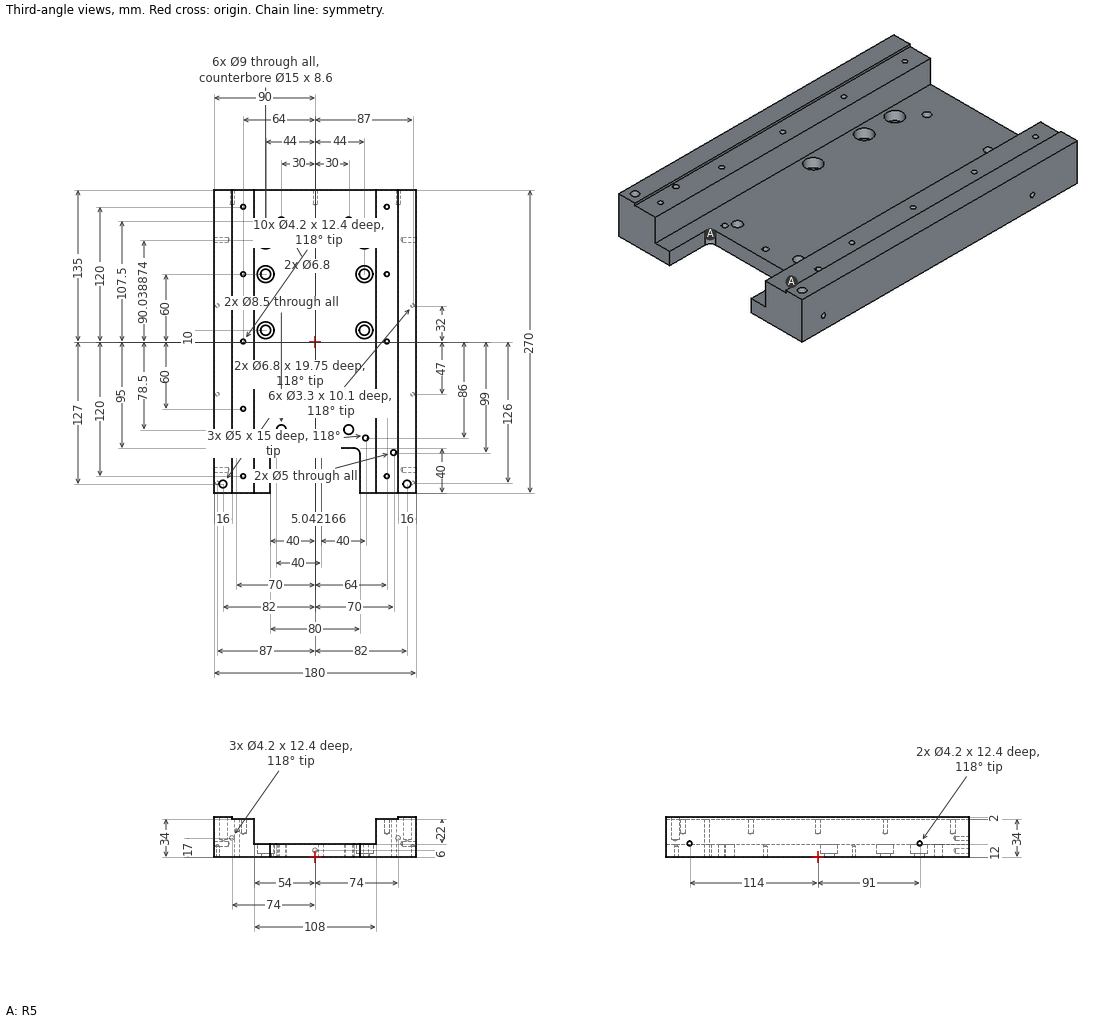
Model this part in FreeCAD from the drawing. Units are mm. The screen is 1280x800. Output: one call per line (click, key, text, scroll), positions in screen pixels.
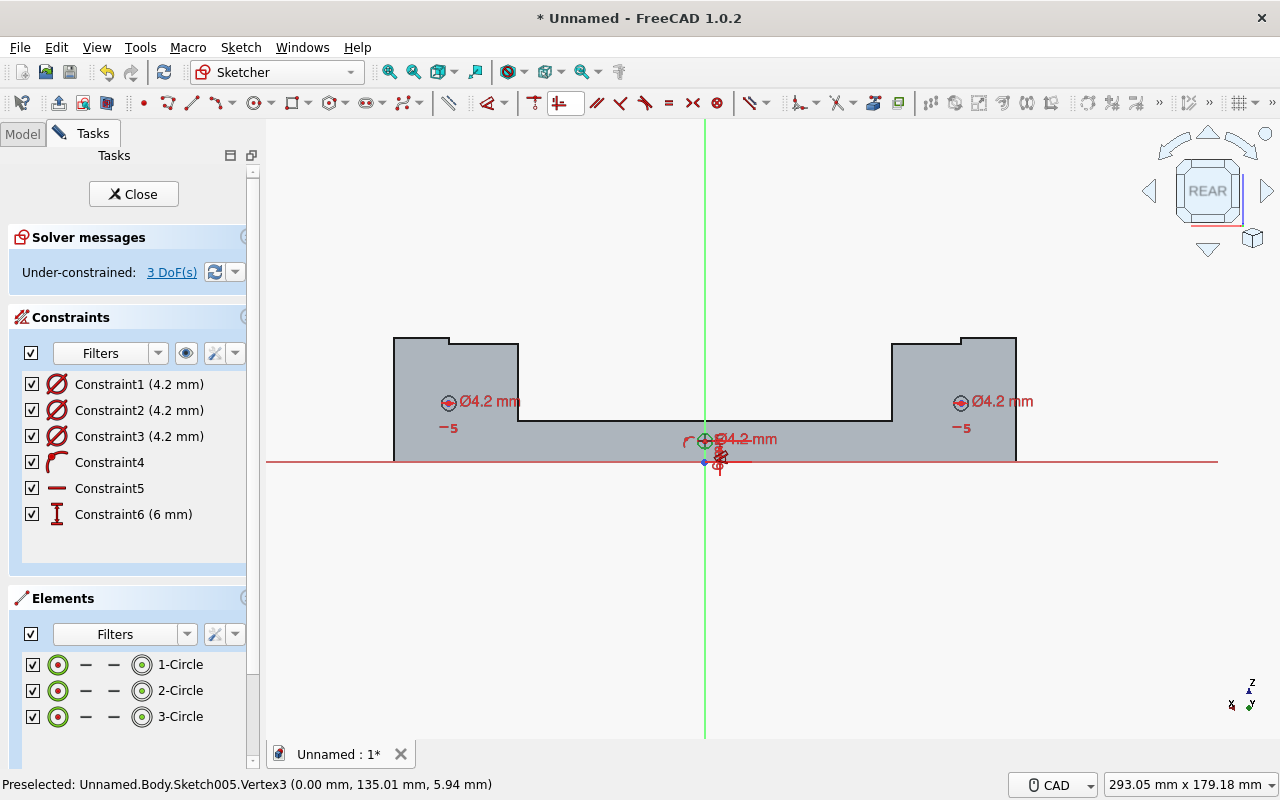
click(961, 403)
click(833, 496)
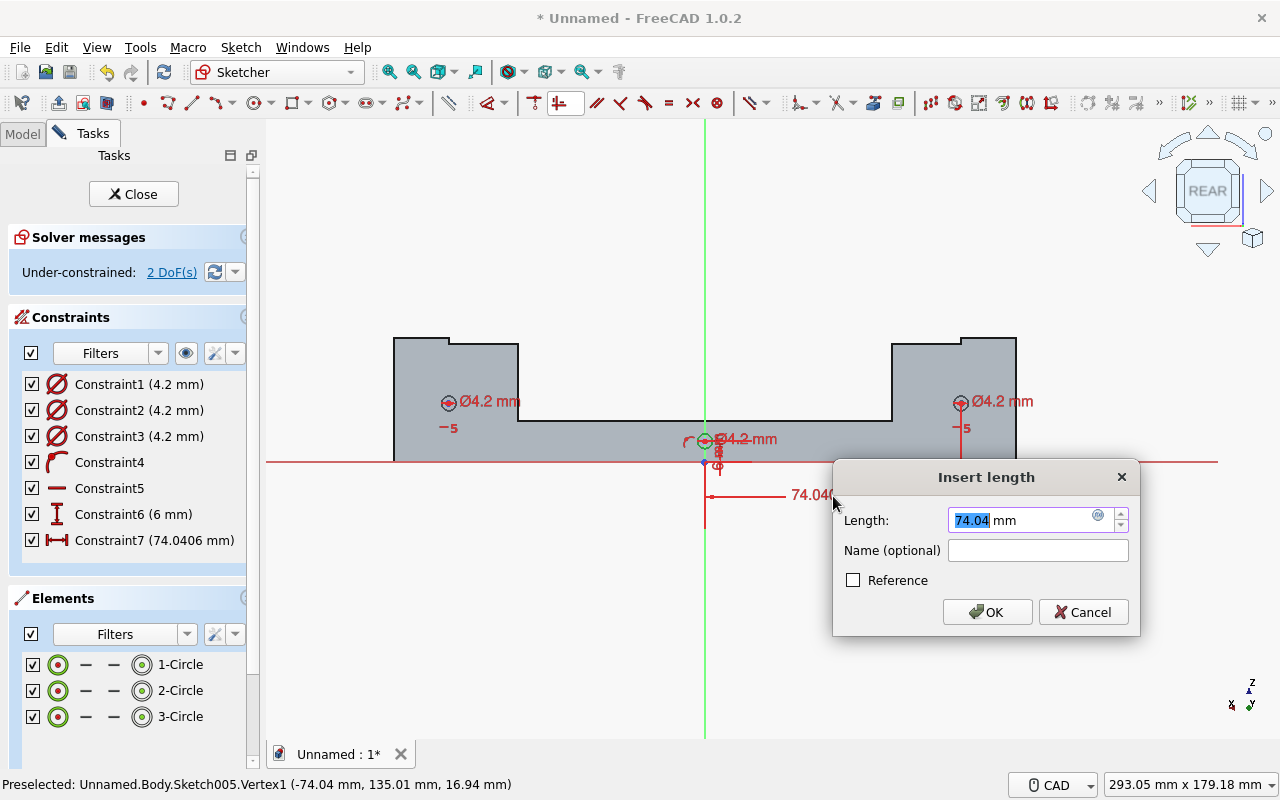
text(74)
key(Return)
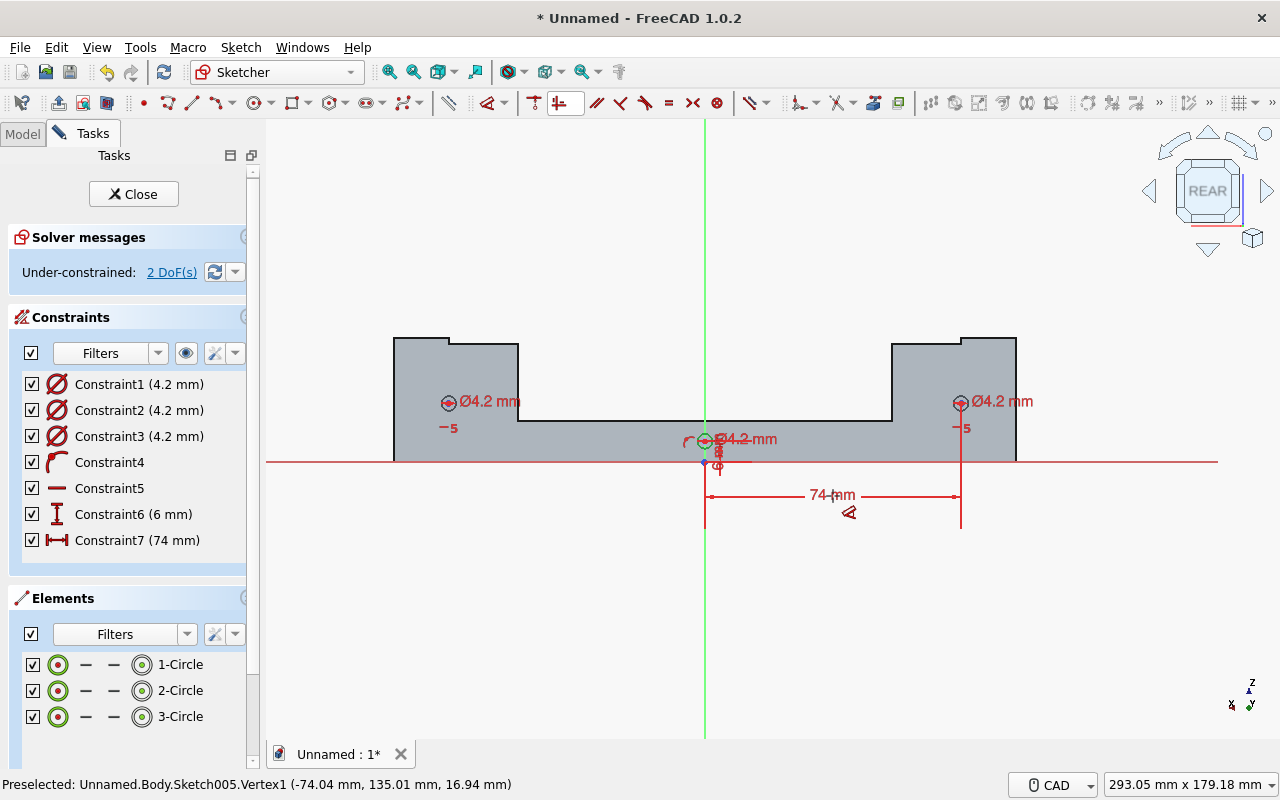
click(961, 403)
click(995, 433)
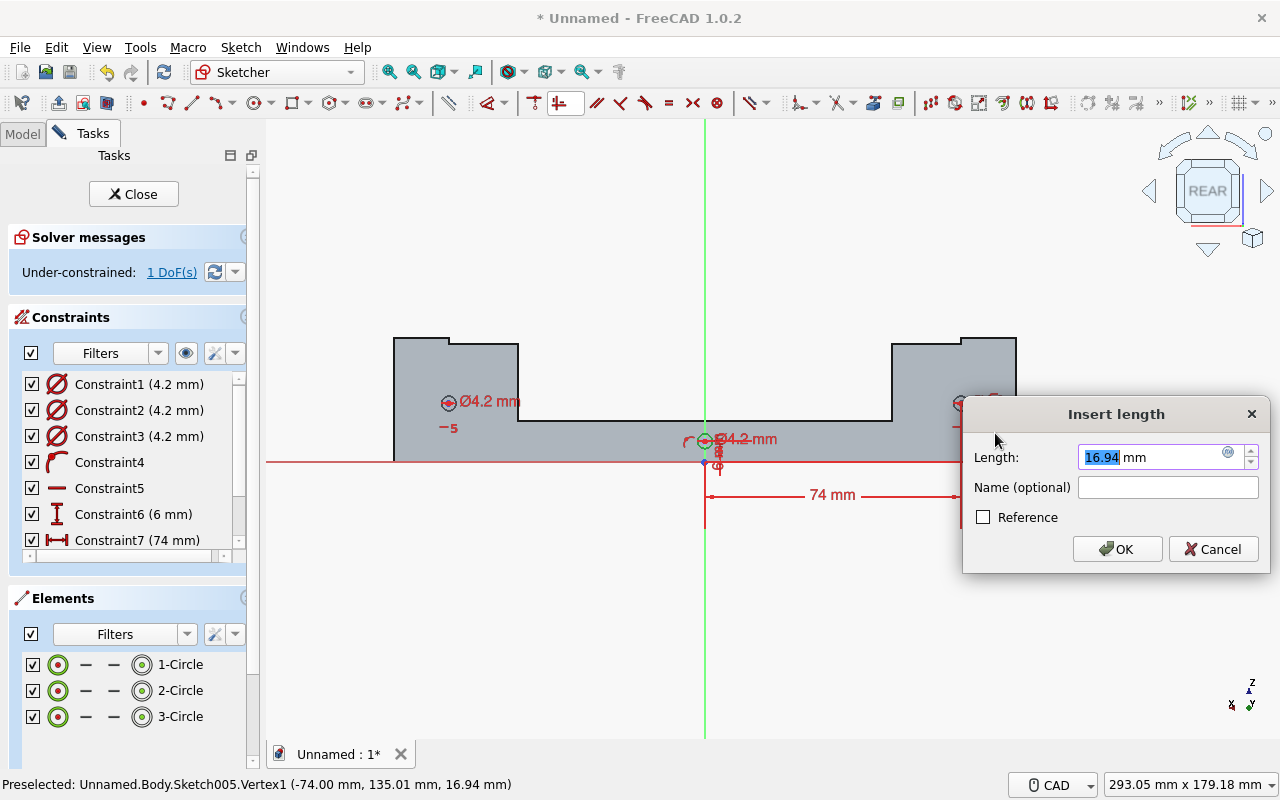
text(17)
key(Return)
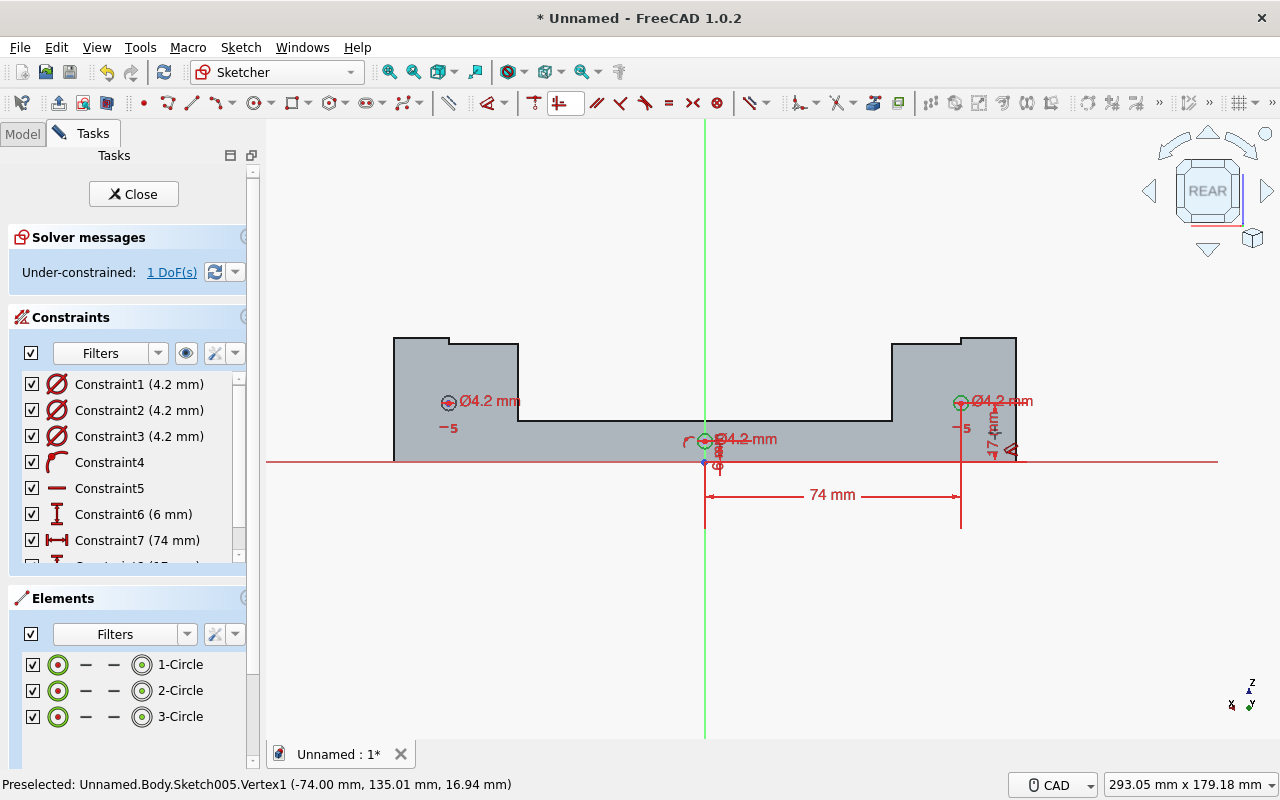
click(449, 403)
click(577, 496)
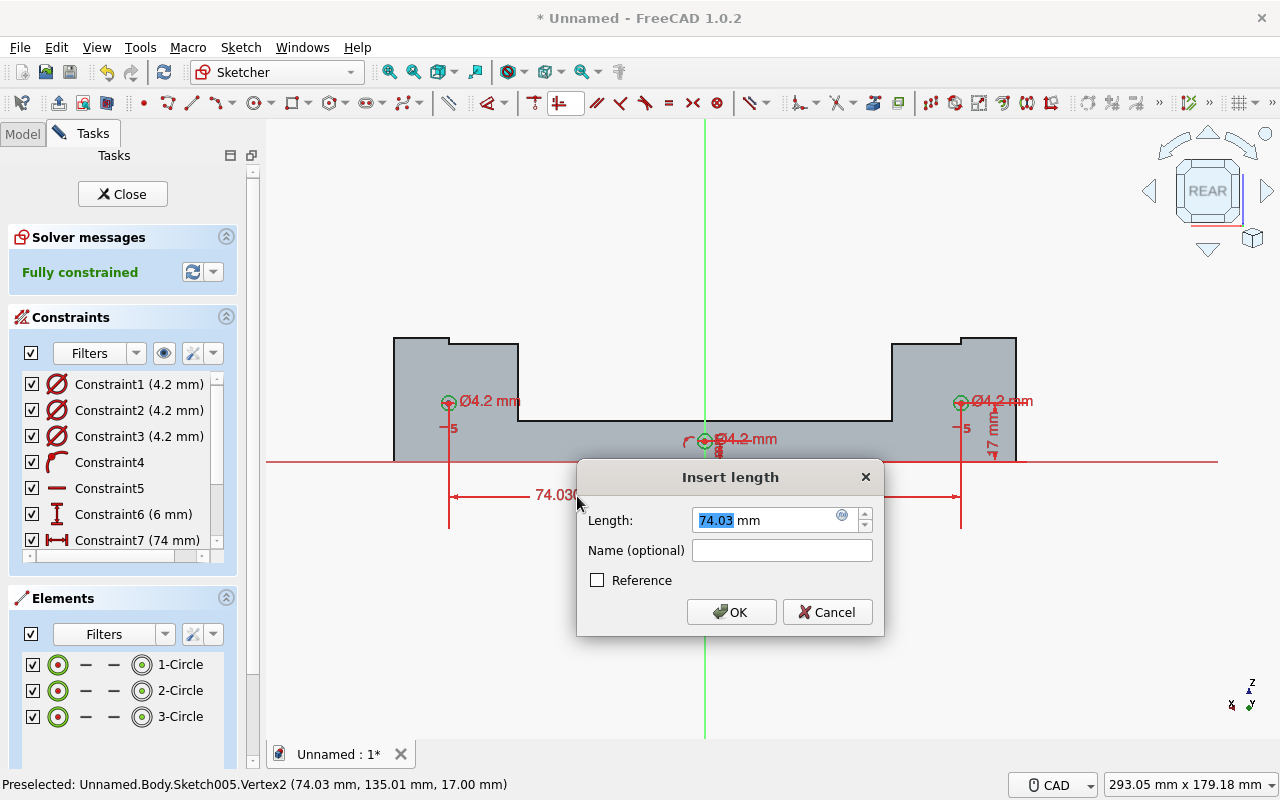
text(74)
key(Return)
key(Escape)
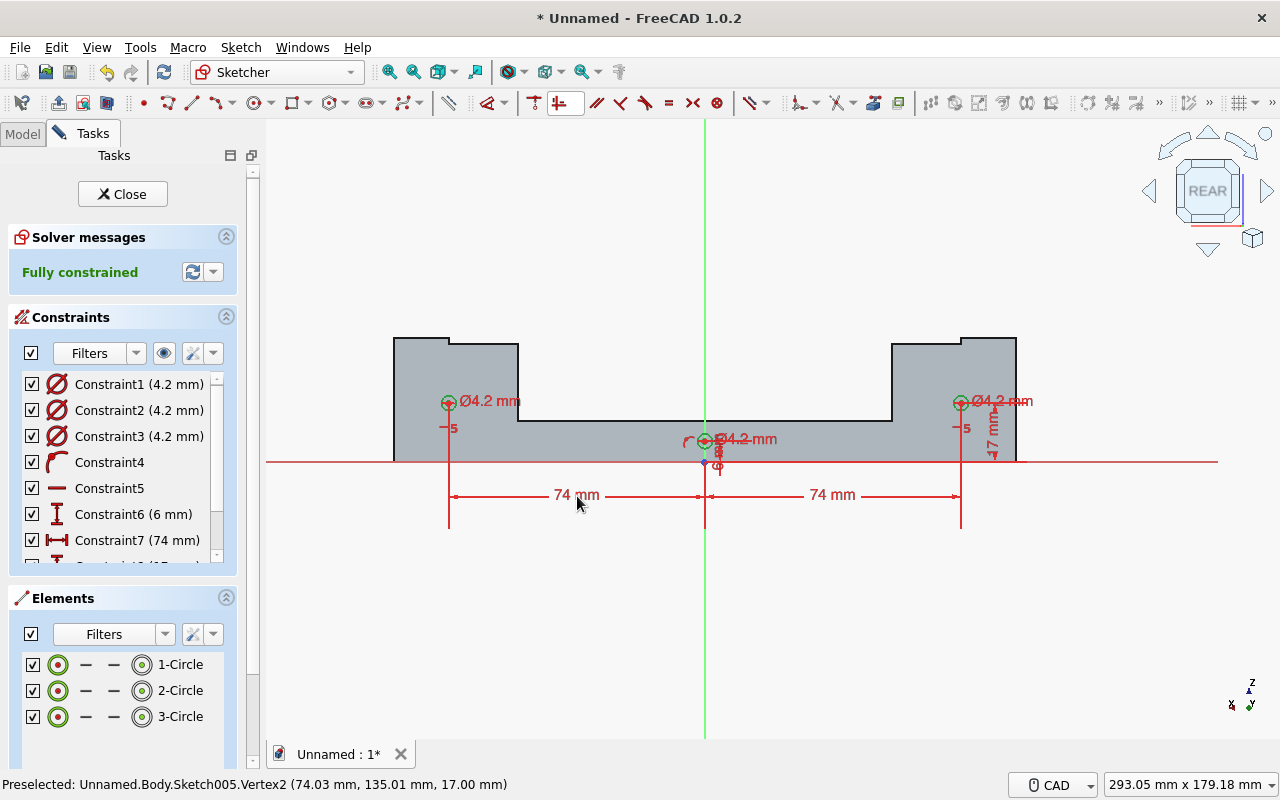
click(123, 194)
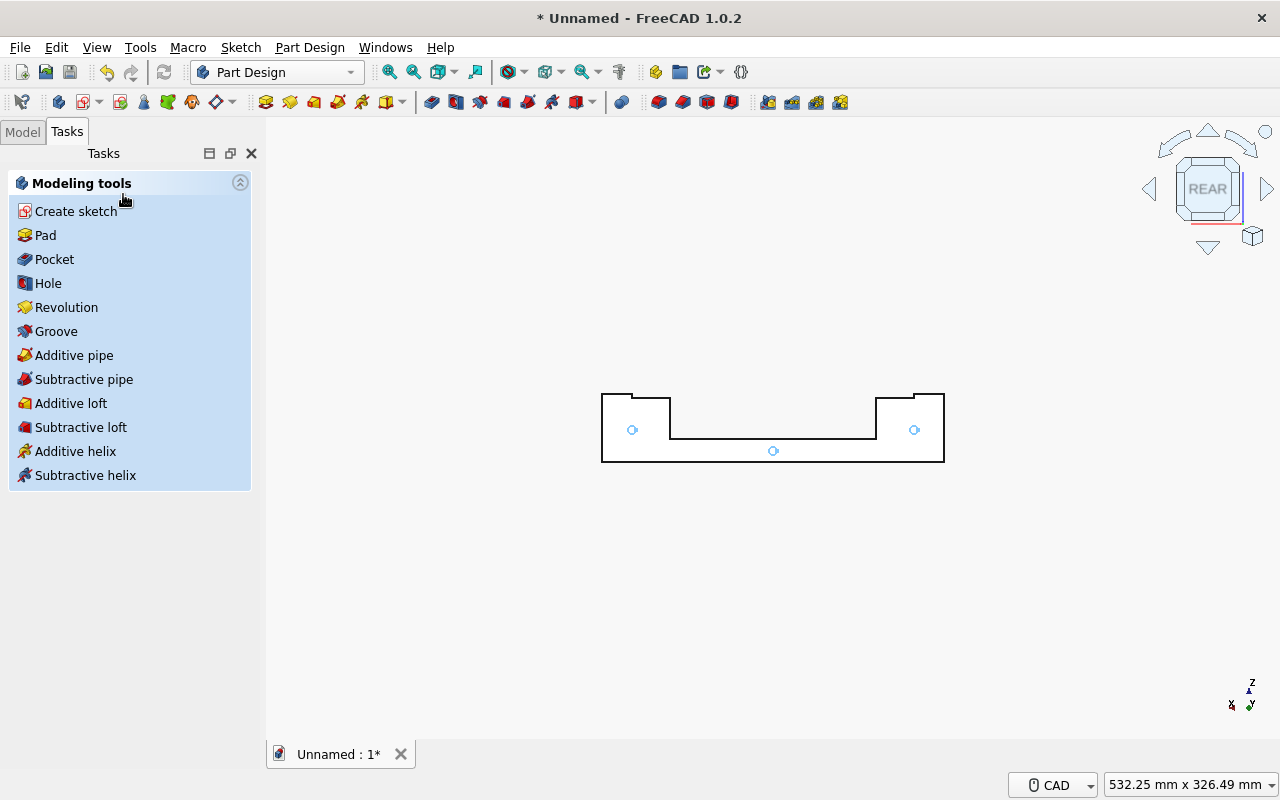
click(456, 102)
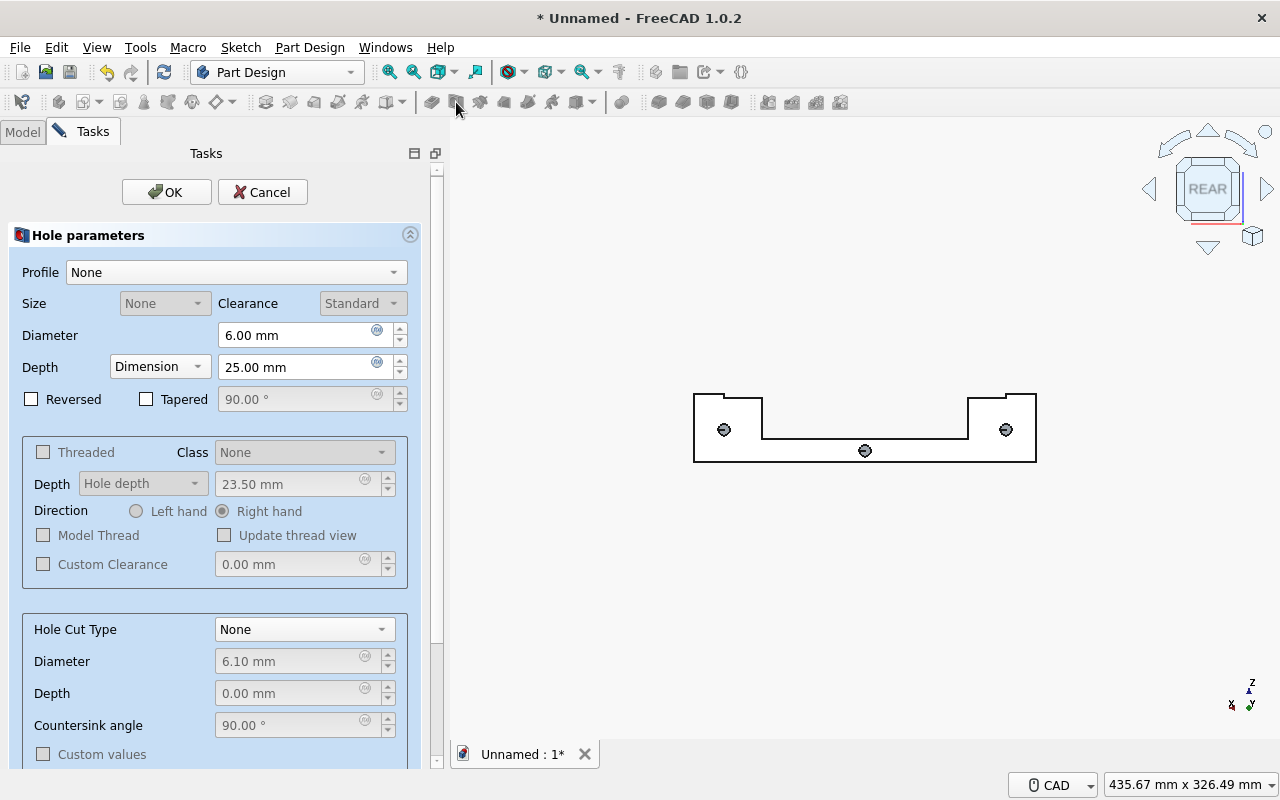
triple_click(305, 335)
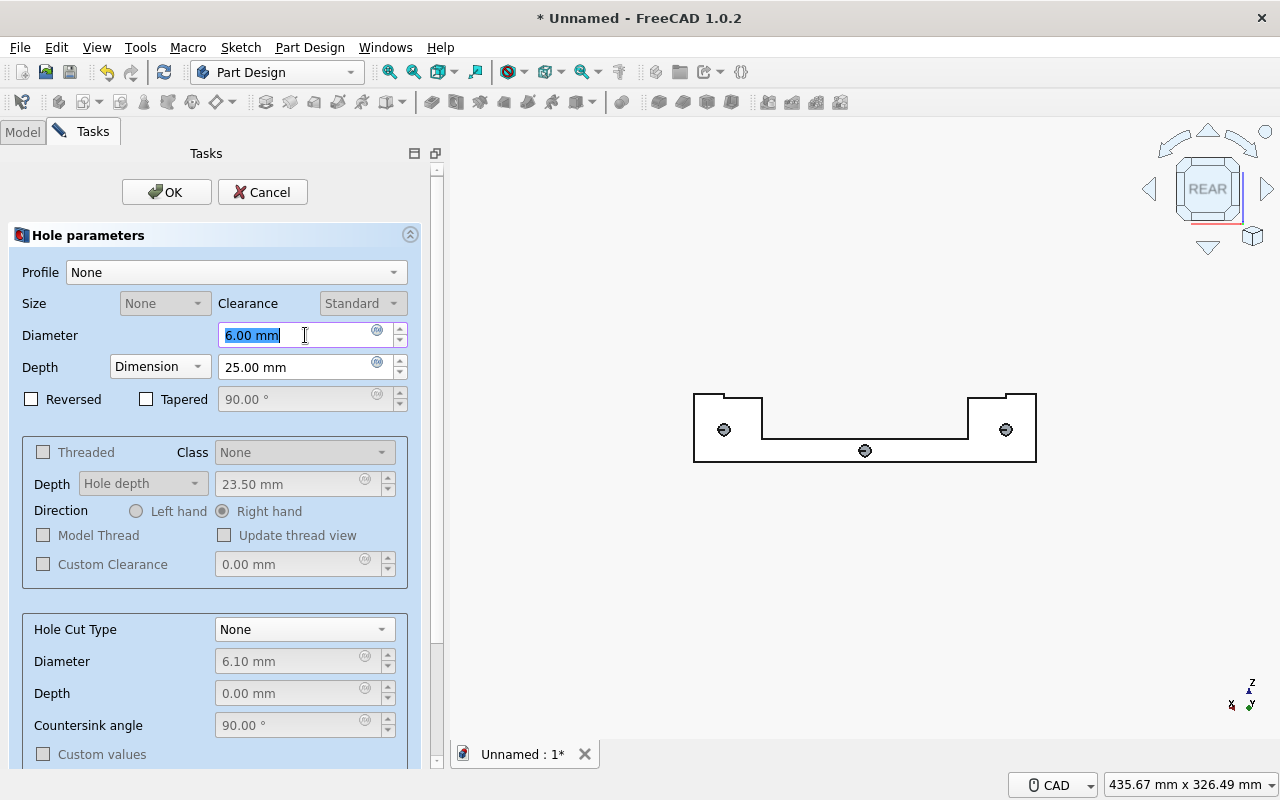
text(4.2)
key(Tab)